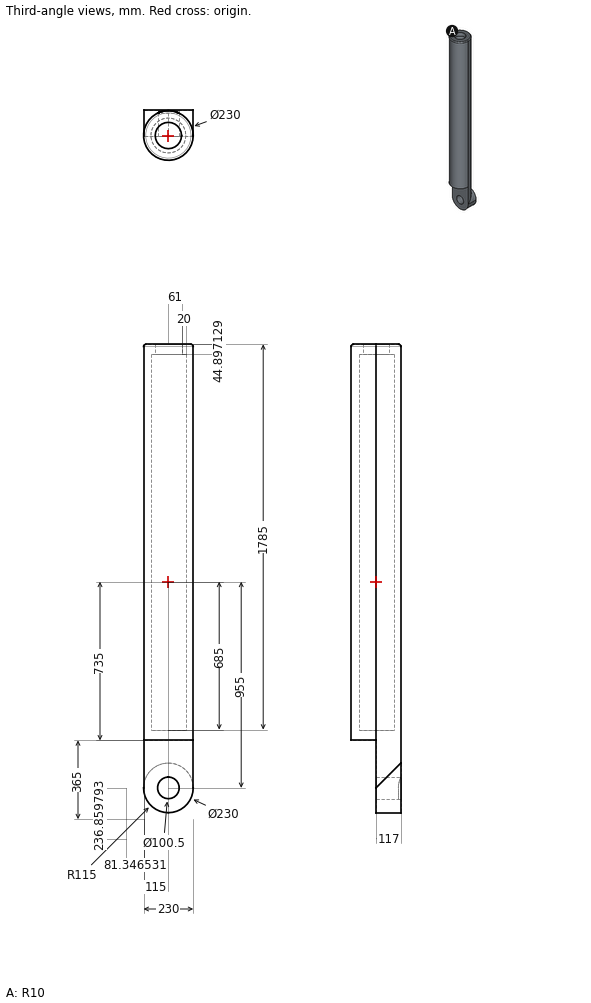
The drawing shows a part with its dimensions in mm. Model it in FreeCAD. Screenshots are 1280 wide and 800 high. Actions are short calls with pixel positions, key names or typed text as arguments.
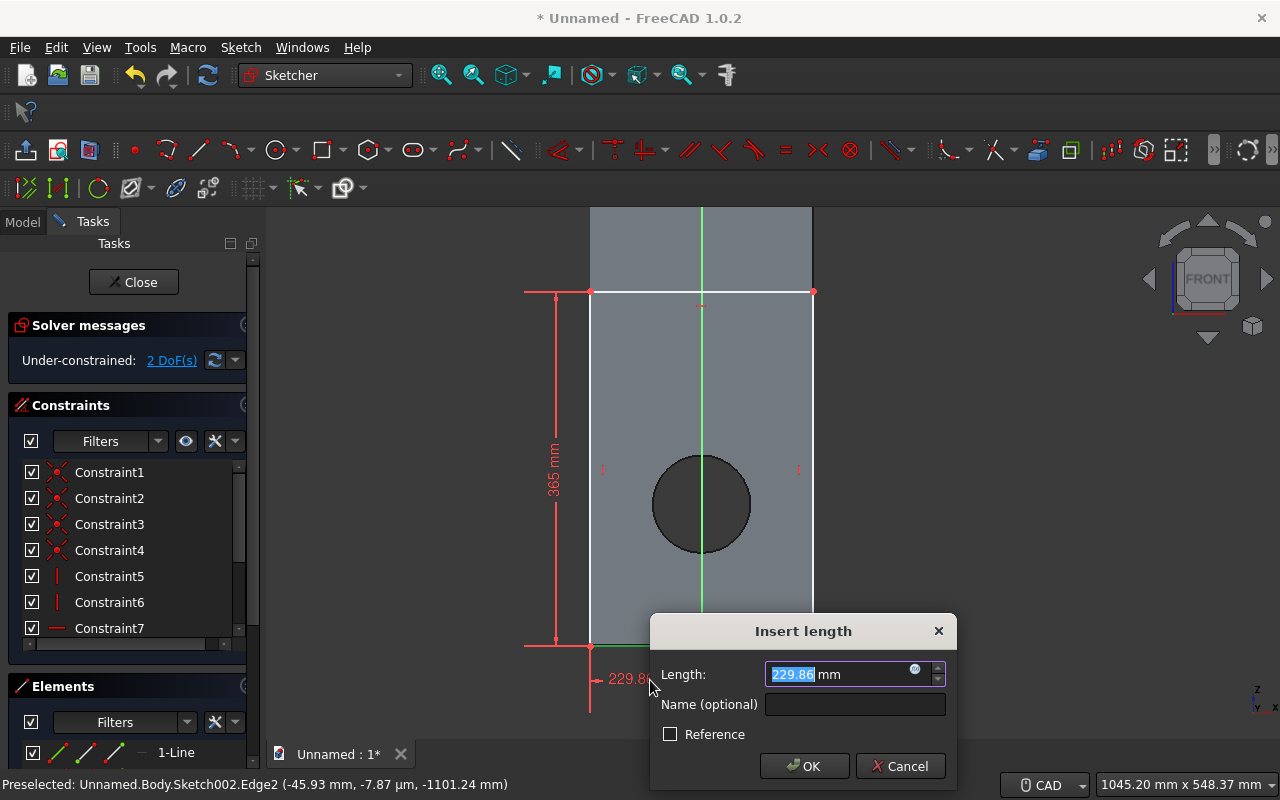
text(230)
key(Return)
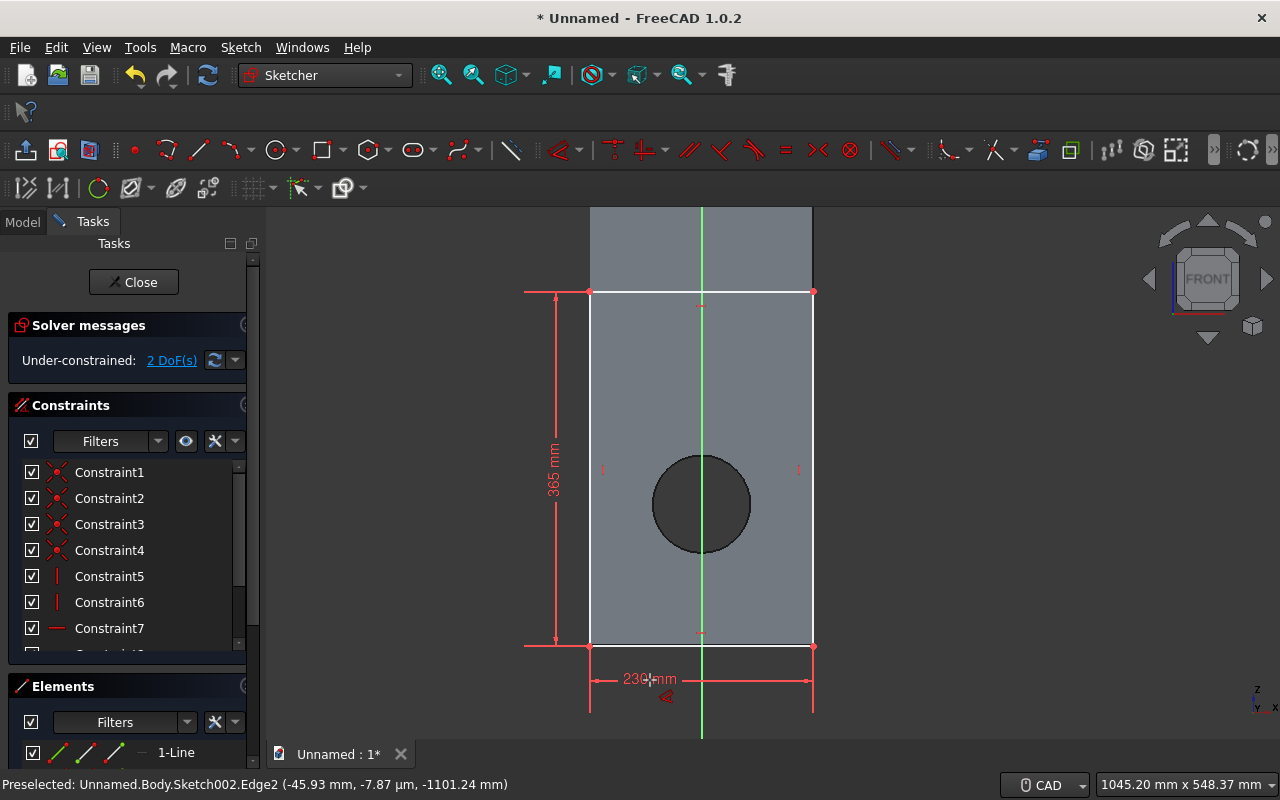
click(590, 292)
click(646, 326)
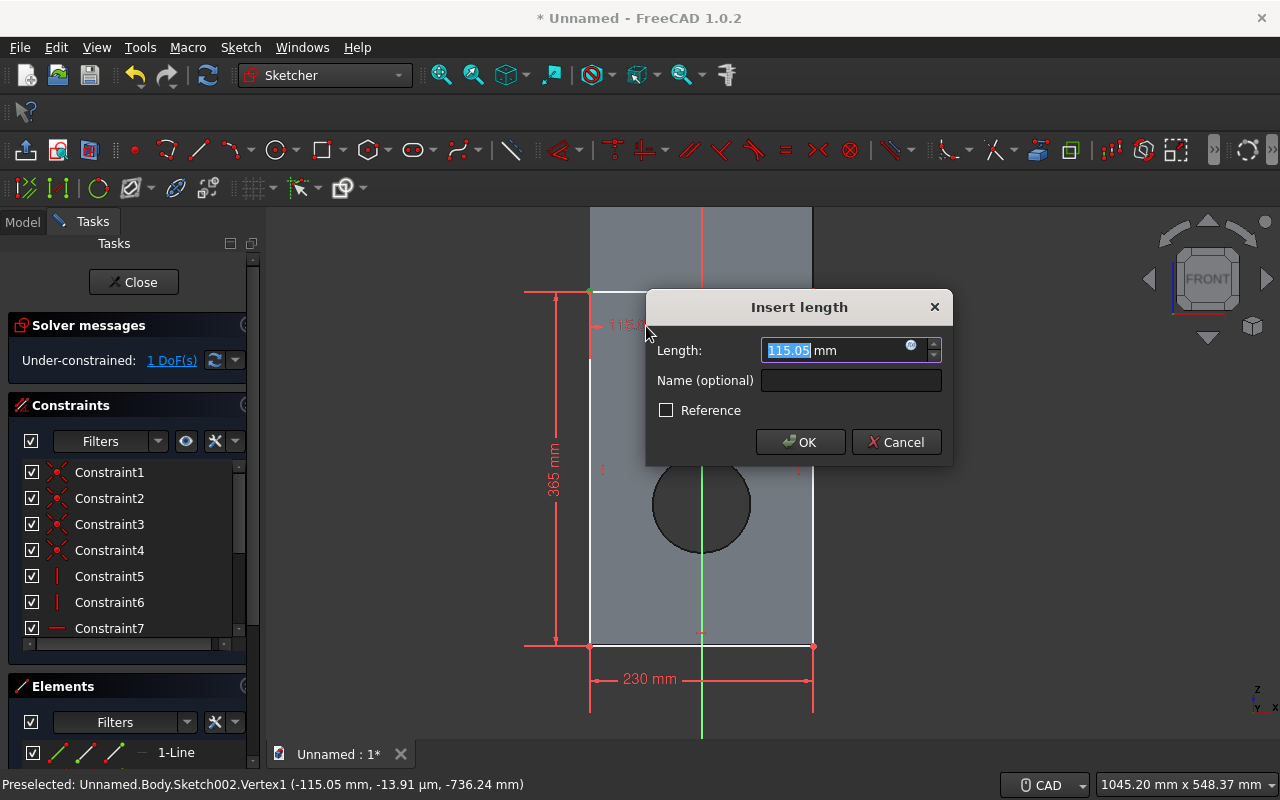
text(115)
key(Return)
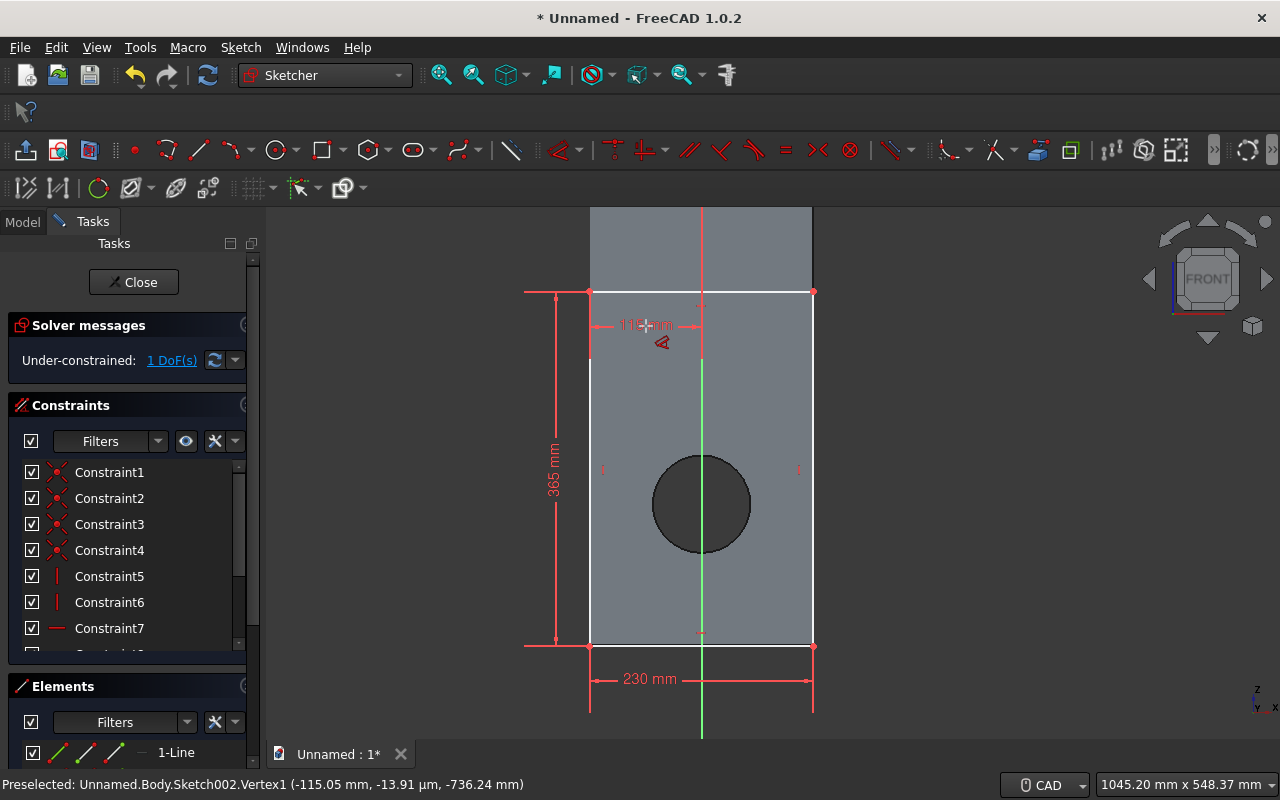
click(590, 292)
click(556, 263)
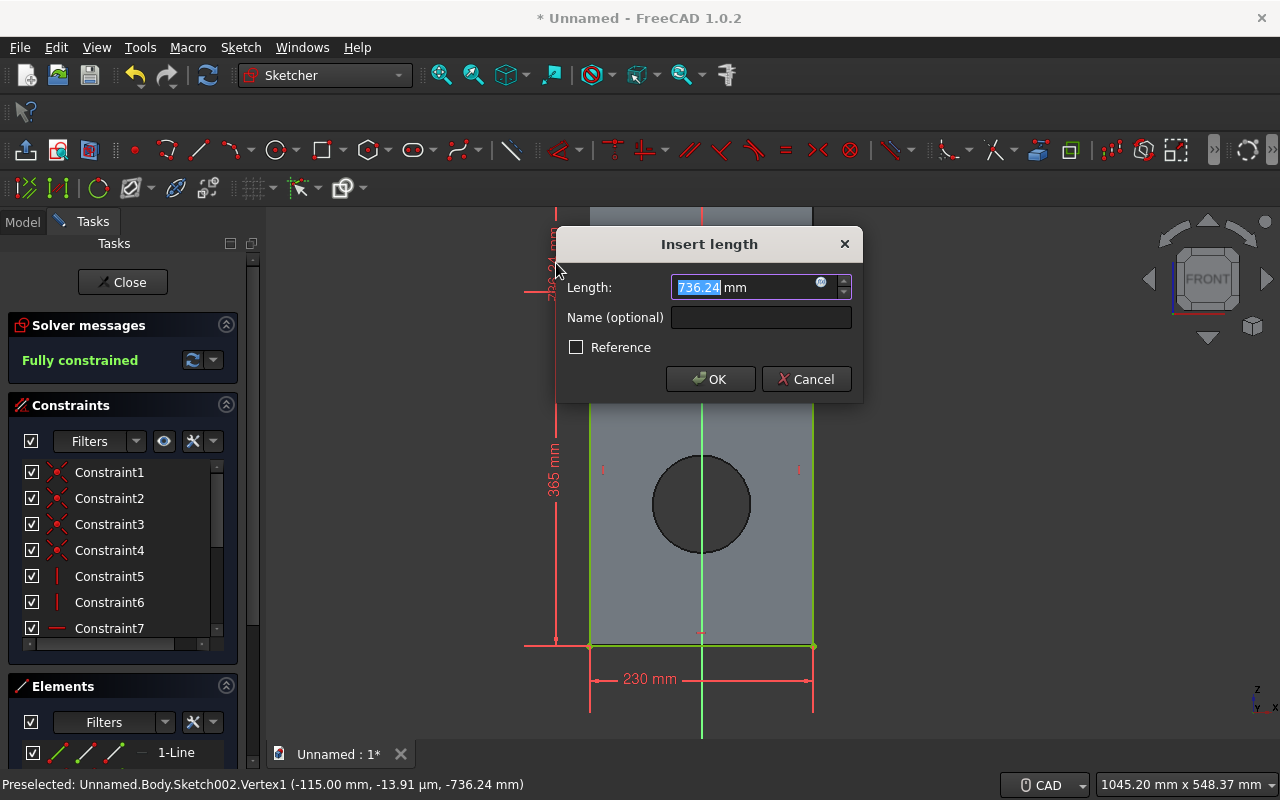
text(735)
key(Return)
key(Escape)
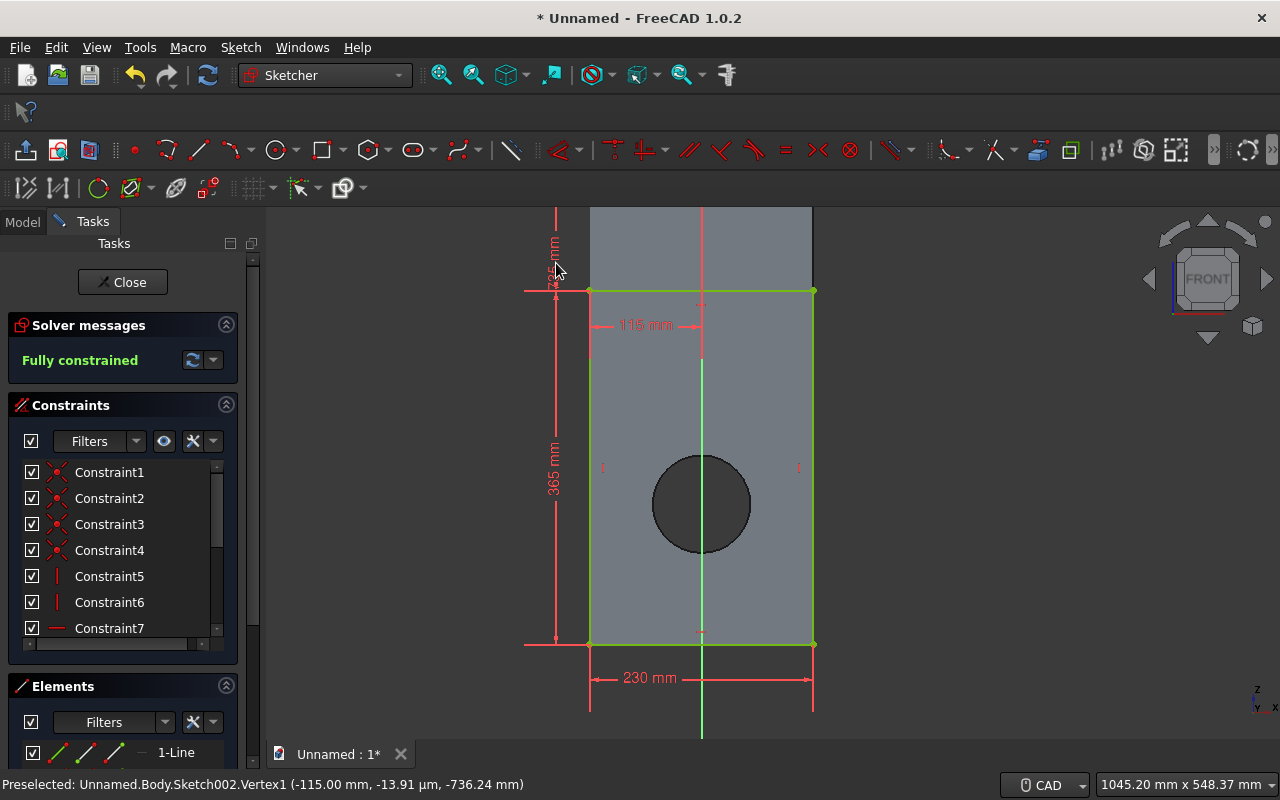
click(123, 282)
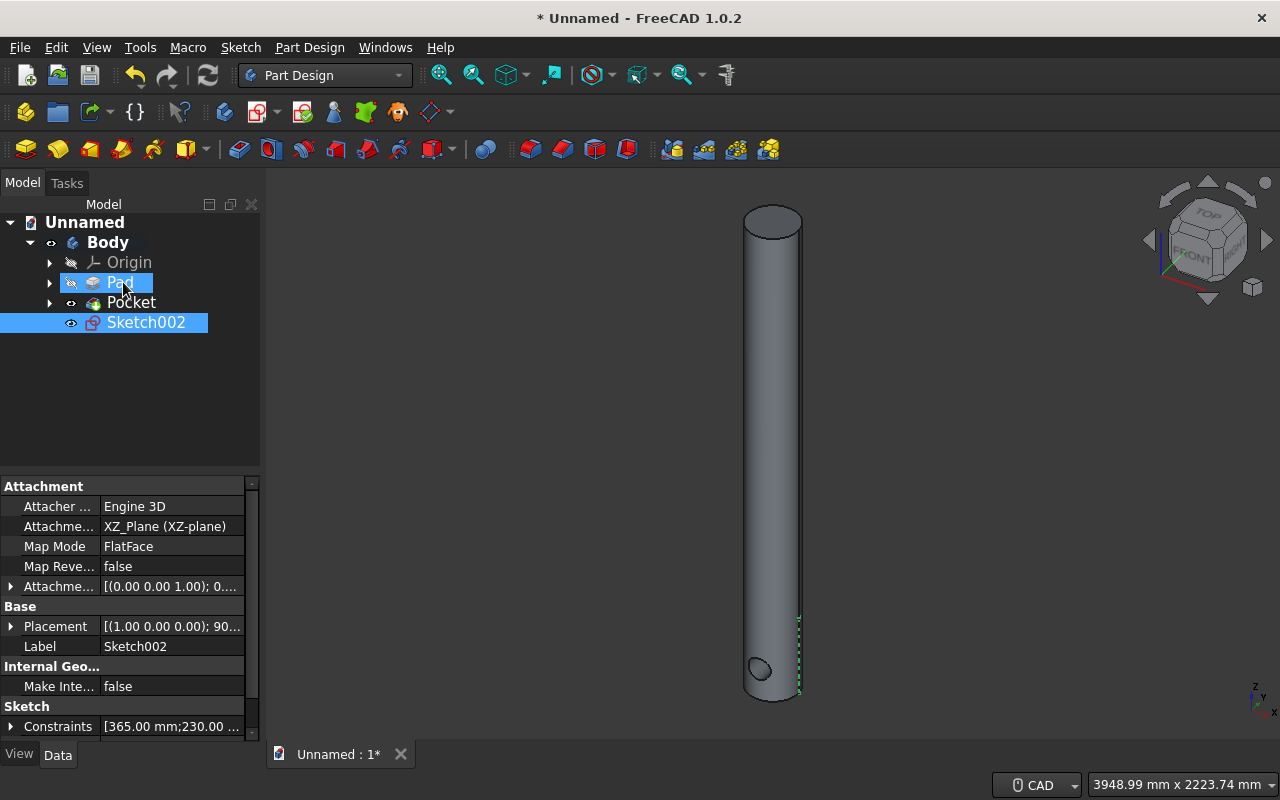
click(240, 150)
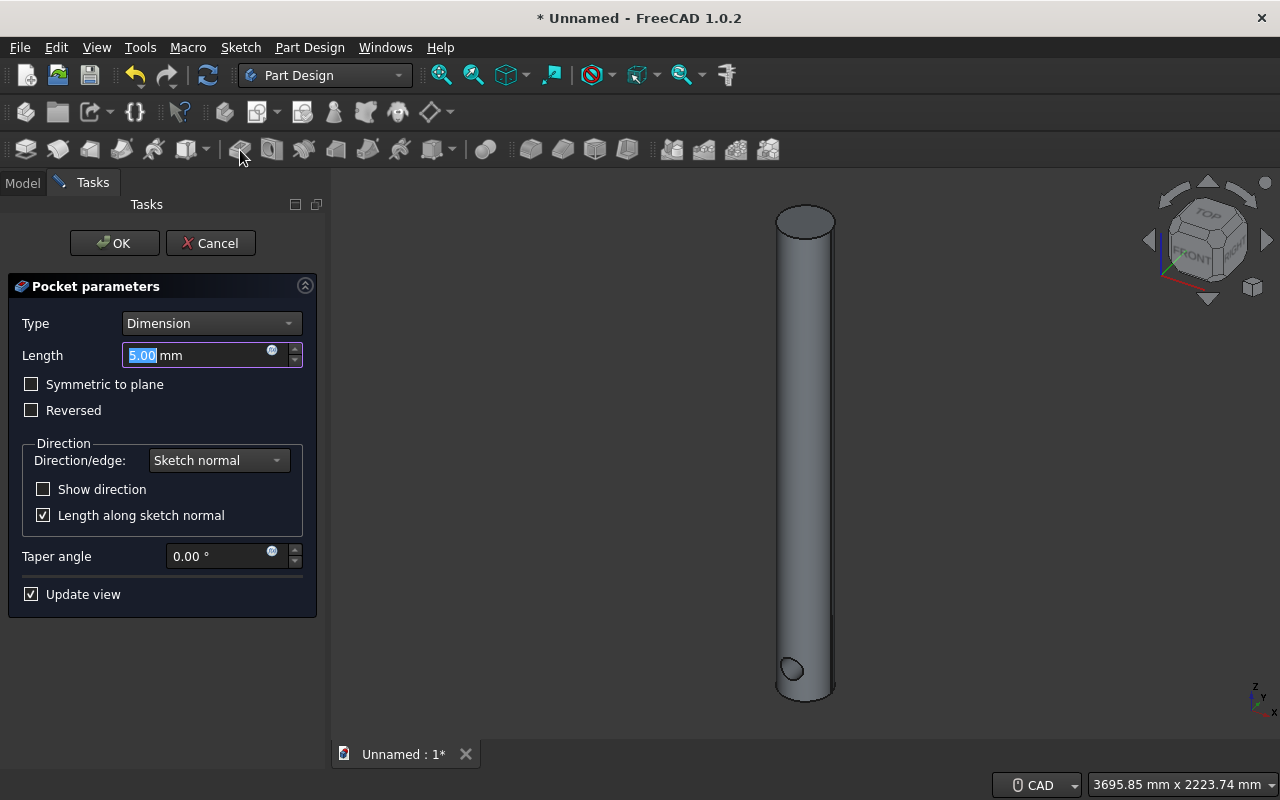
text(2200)
key(Tab)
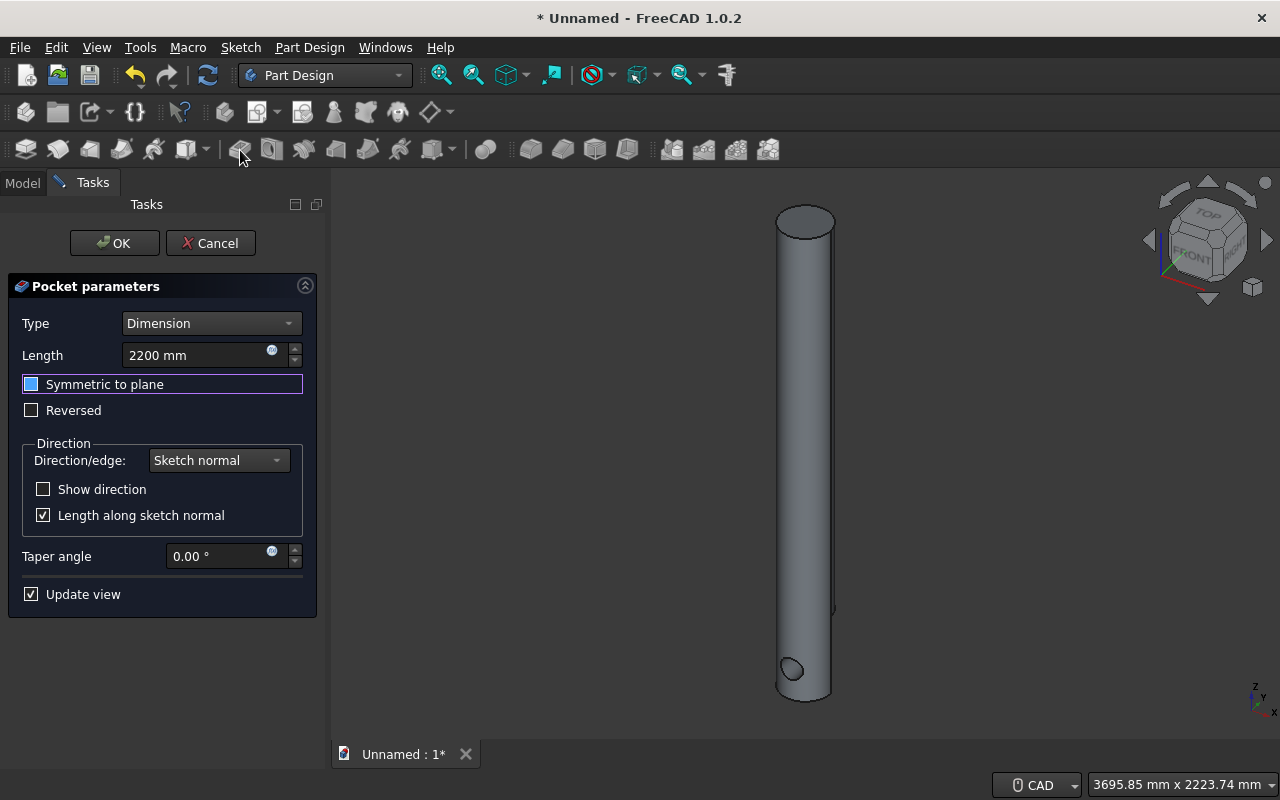
click(30, 410)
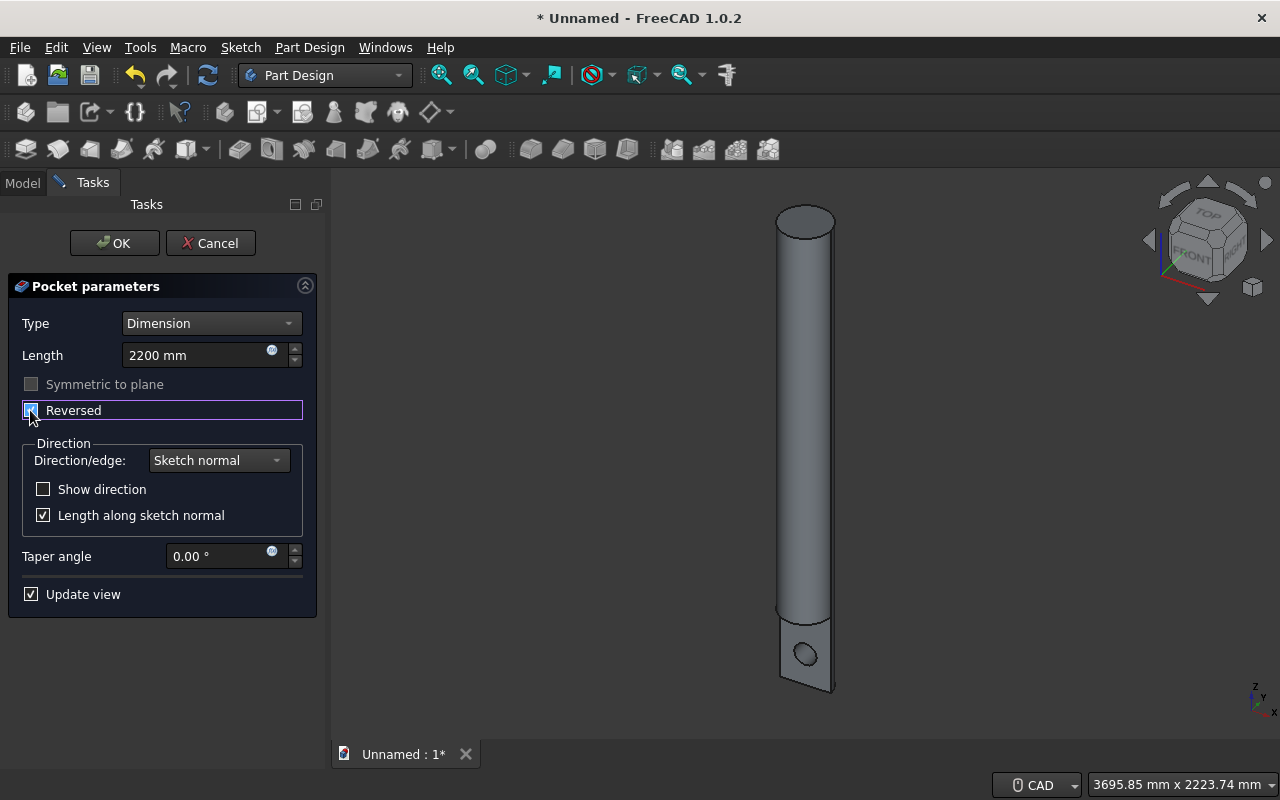
click(115, 243)